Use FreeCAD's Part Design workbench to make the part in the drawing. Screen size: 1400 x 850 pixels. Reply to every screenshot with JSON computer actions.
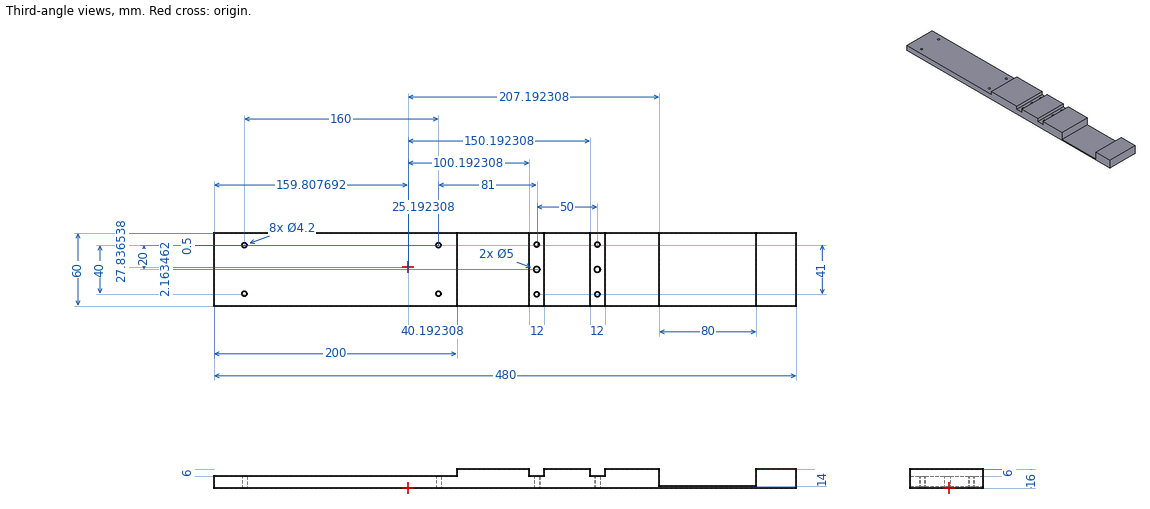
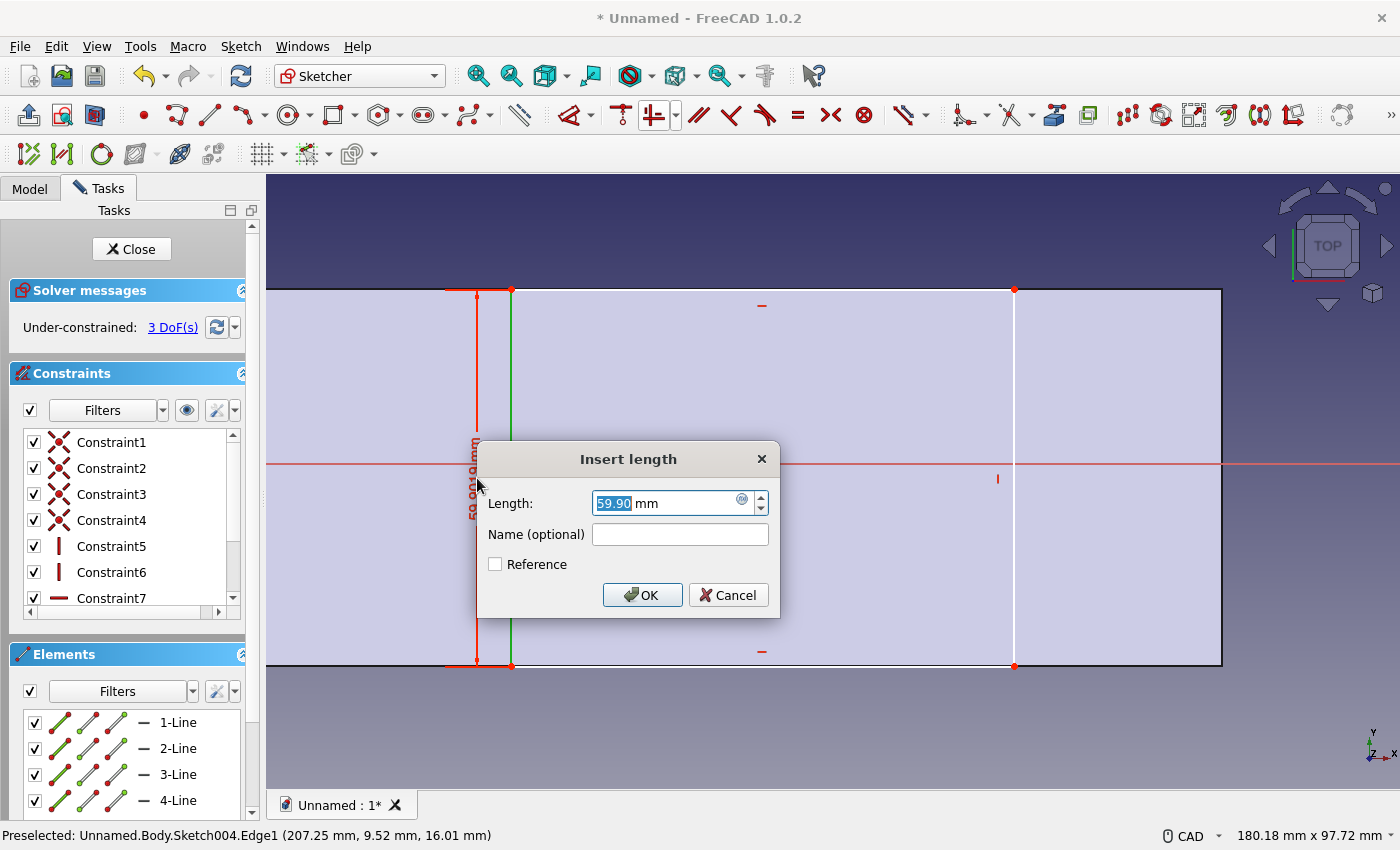
{"action": "type", "text": "60"}
{"action": "key", "text": "Return"}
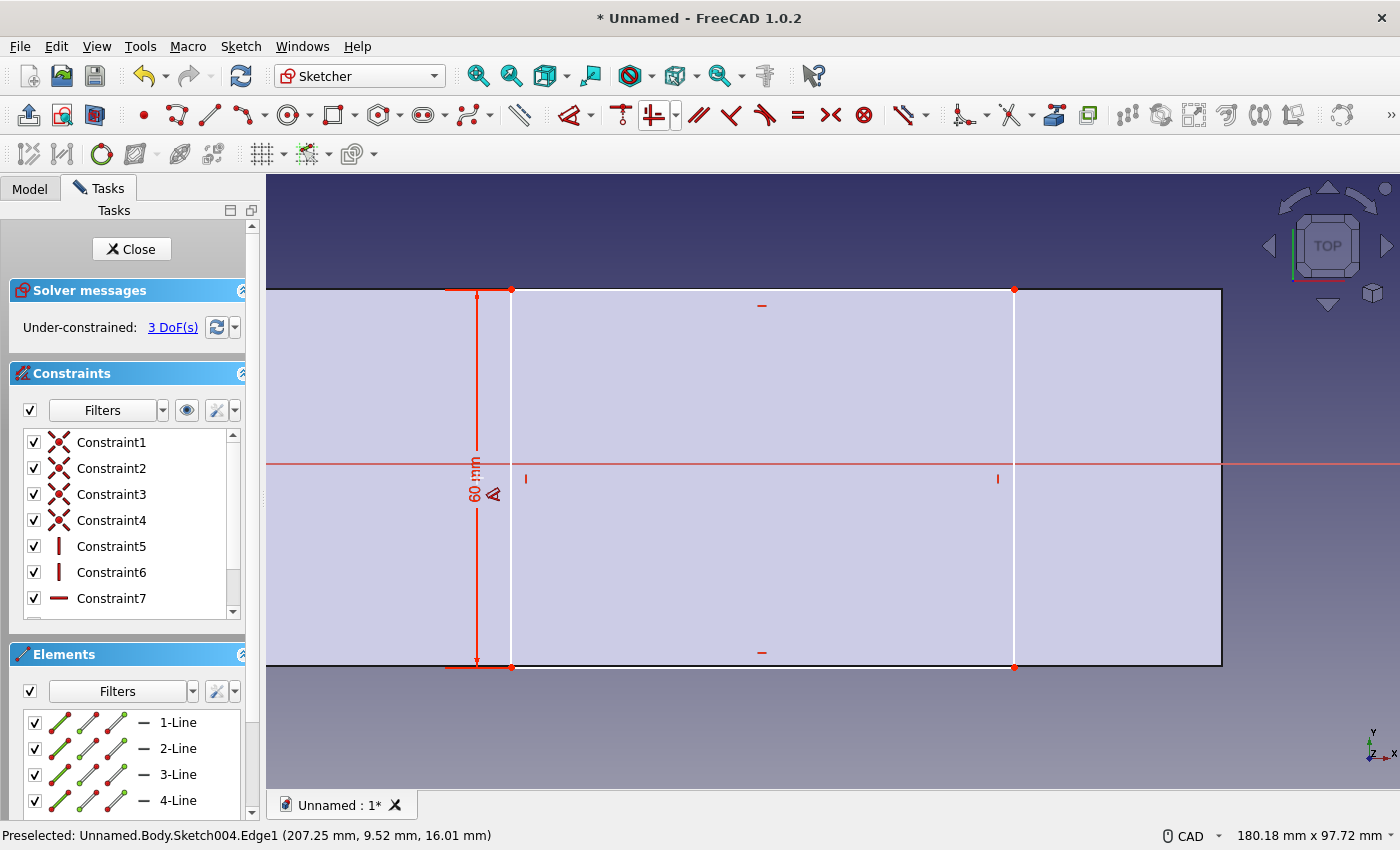
{"action": "left_click", "coordinate": [662, 668]}
{"action": "left_click", "coordinate": [762, 702]}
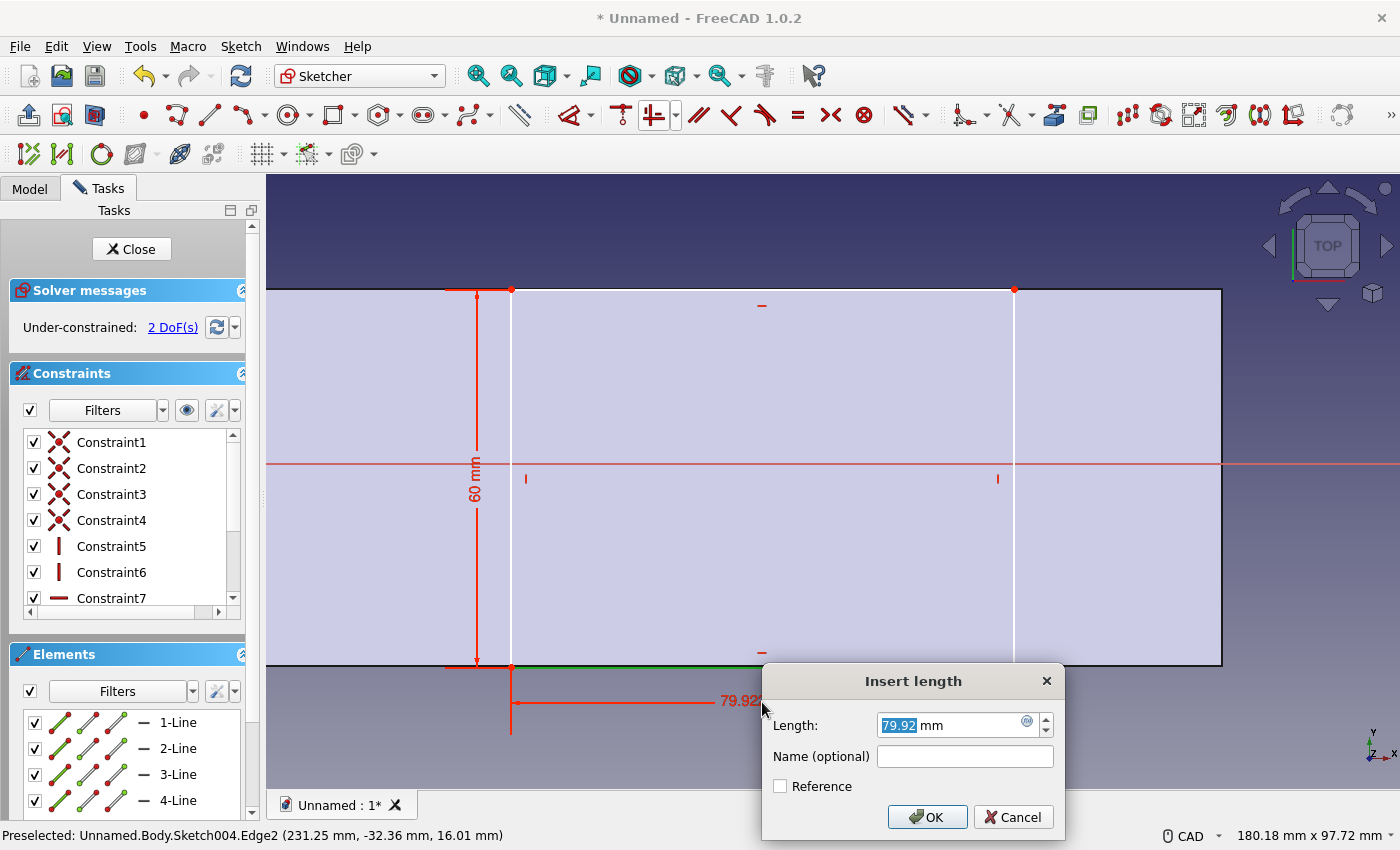
{"action": "type", "text": "80"}
{"action": "key", "text": "Return"}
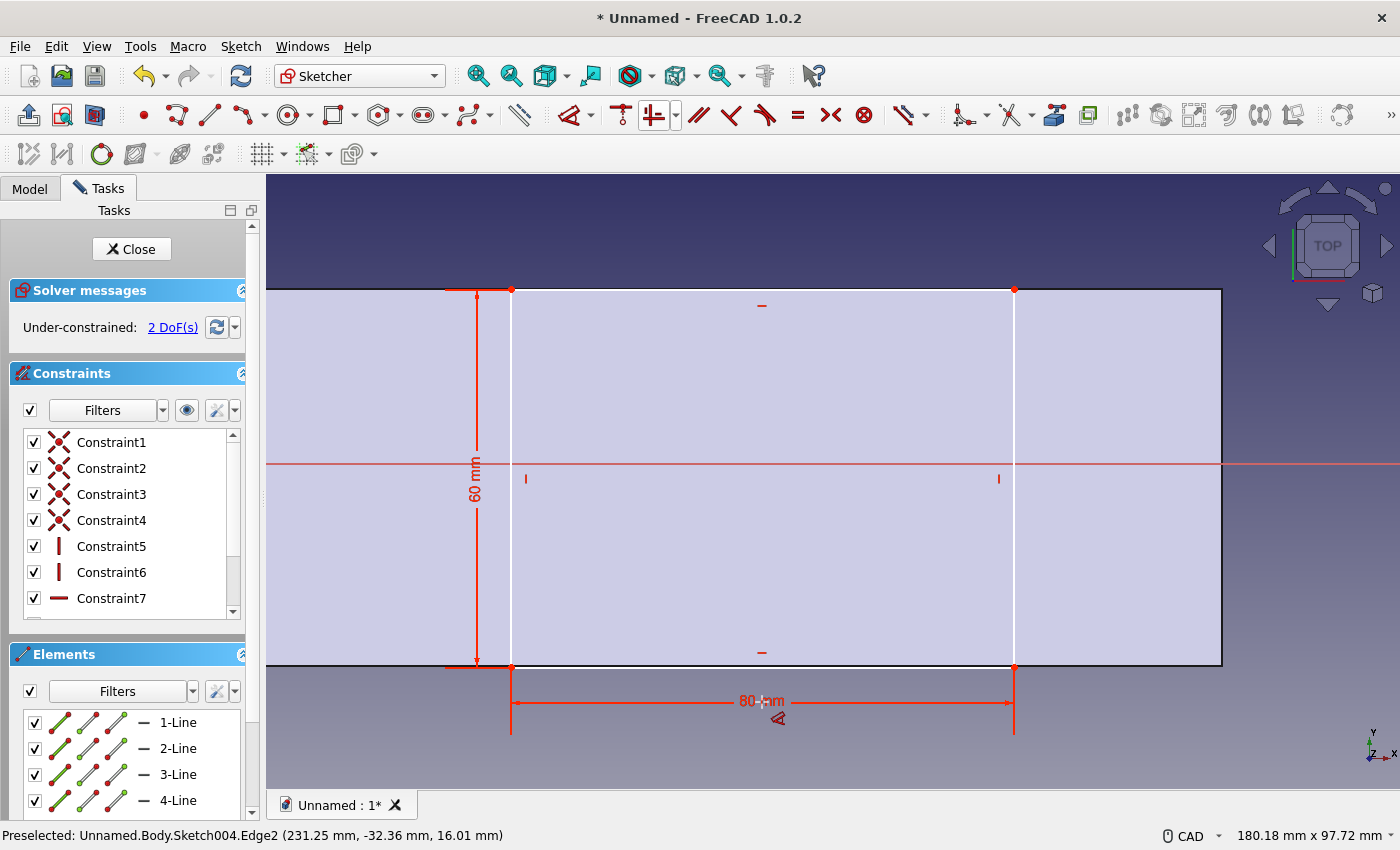
{"action": "left_click", "coordinate": [511, 290]}
{"action": "left_click", "coordinate": [545, 377]}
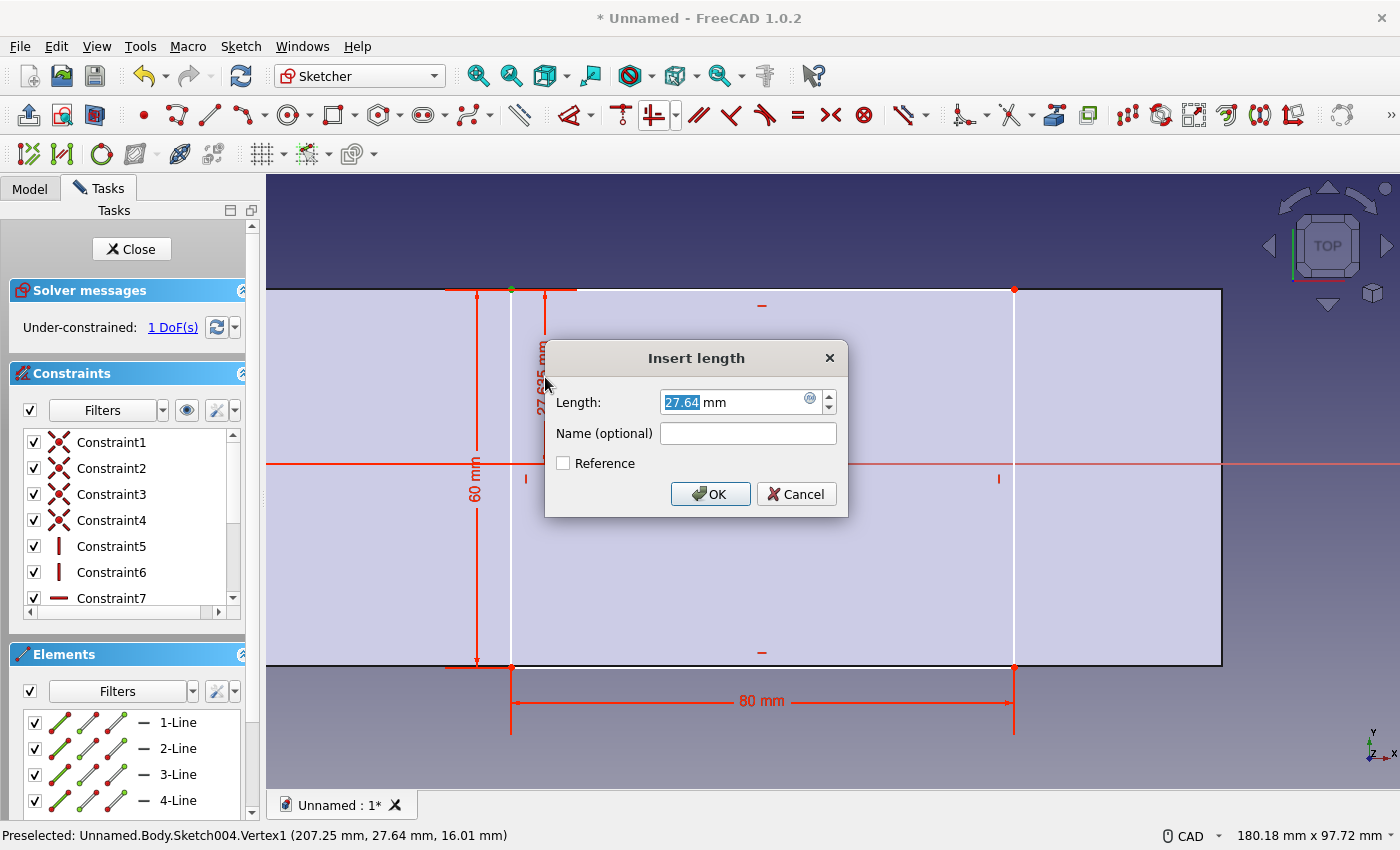
{"action": "type", "text": "27.836538"}
{"action": "key", "text": "Return"}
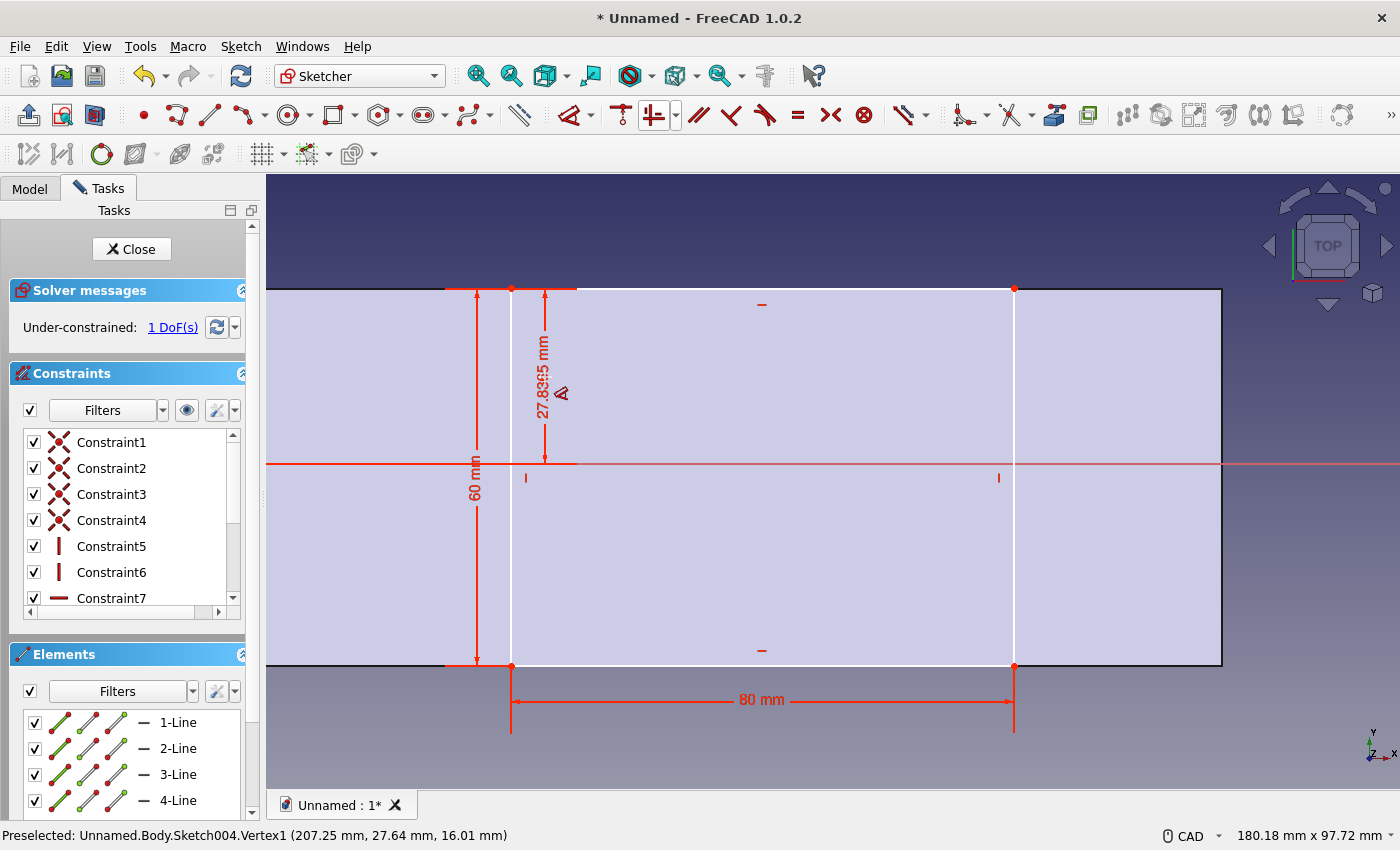
{"action": "left_click", "coordinate": [511, 289]}
{"action": "left_click", "coordinate": [402, 255]}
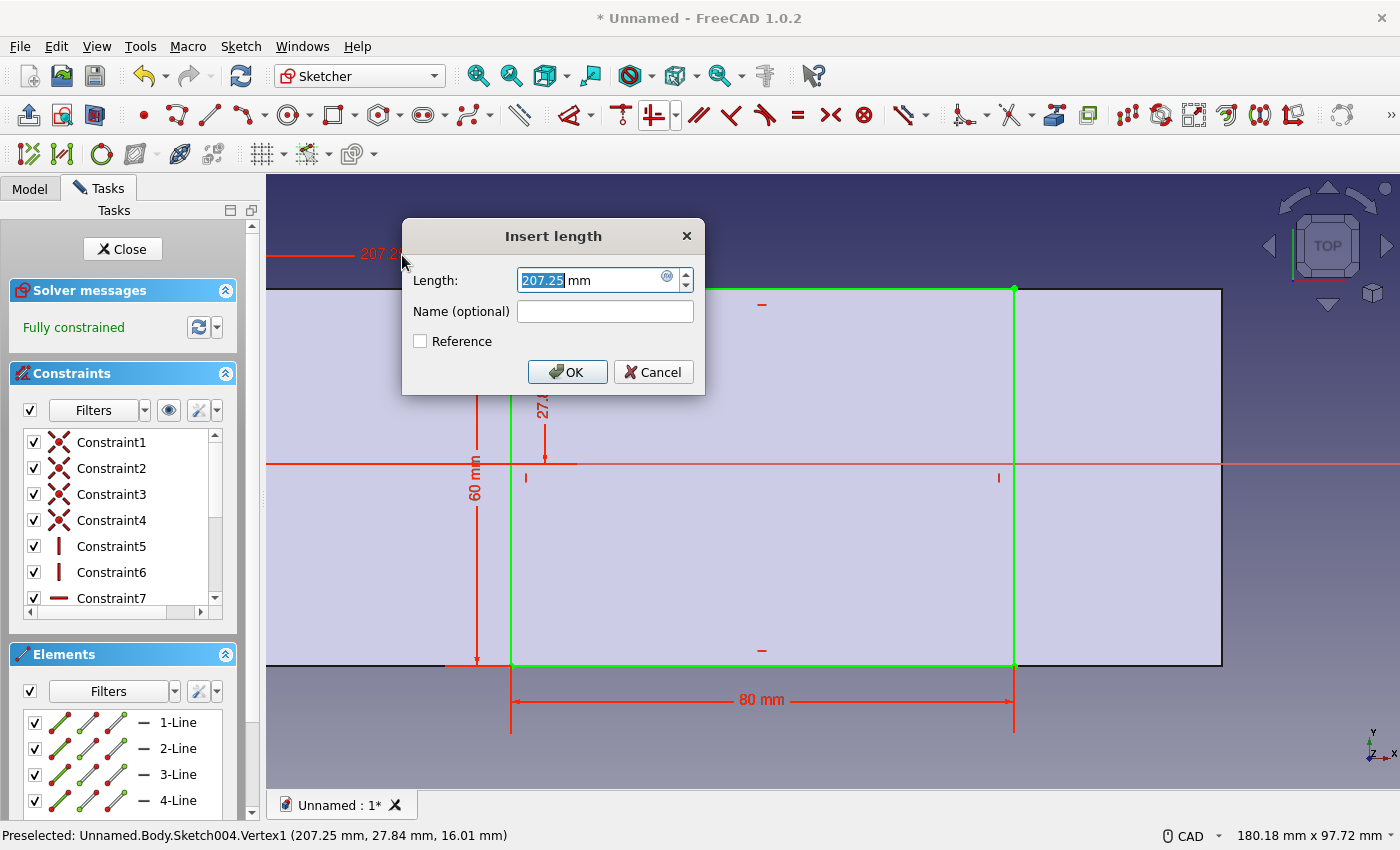
{"action": "type", "text": "207.192308"}
{"action": "key", "text": "Return"}
{"action": "key", "text": "Escape"}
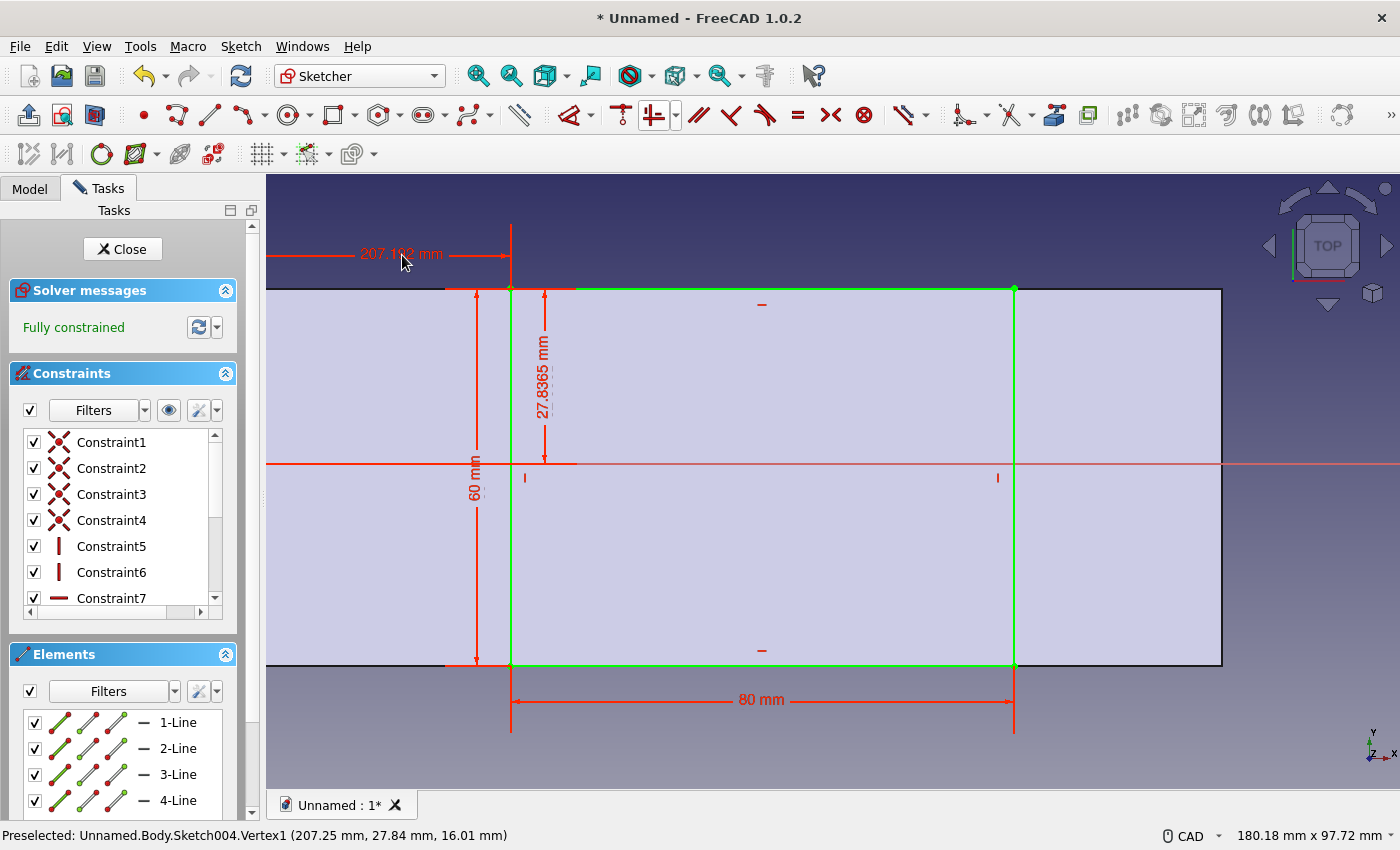
{"action": "left_click", "coordinate": [123, 249]}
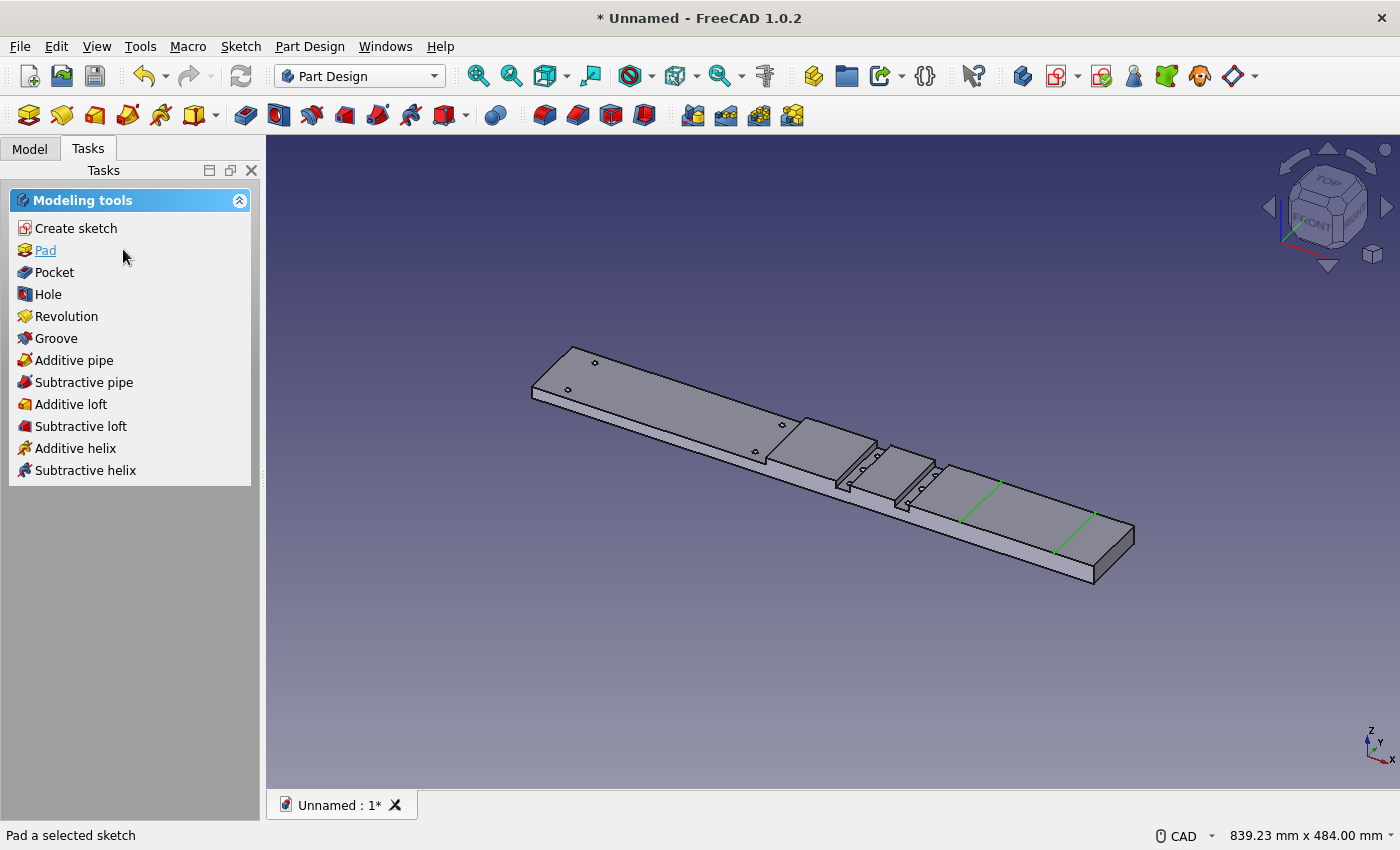
{"action": "left_click", "coordinate": [246, 116]}